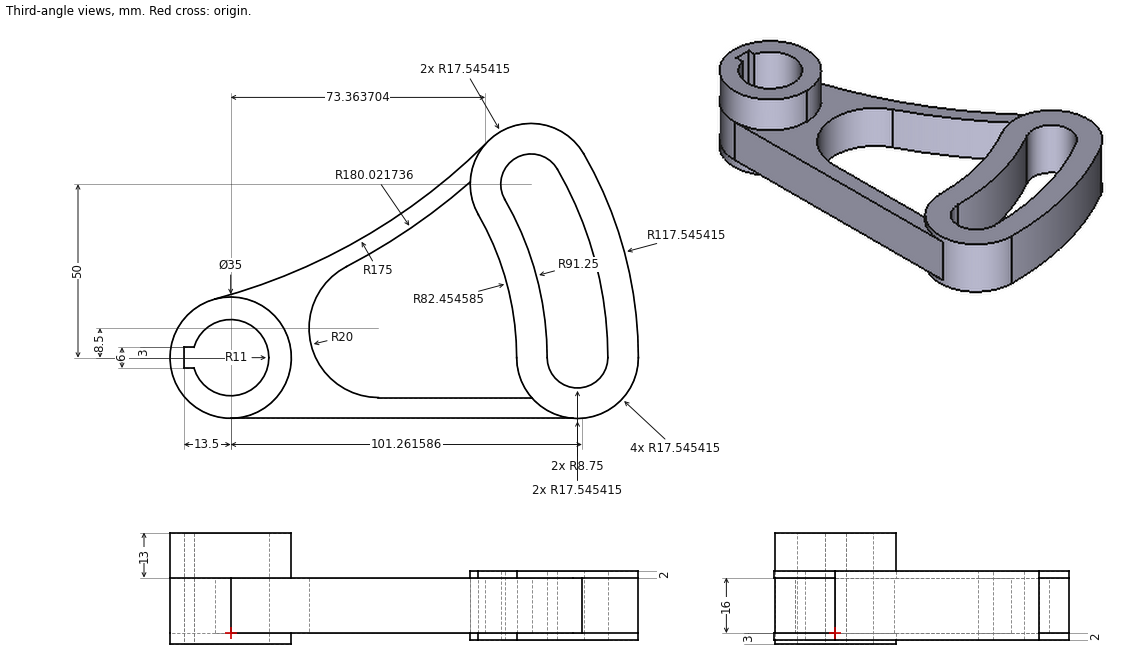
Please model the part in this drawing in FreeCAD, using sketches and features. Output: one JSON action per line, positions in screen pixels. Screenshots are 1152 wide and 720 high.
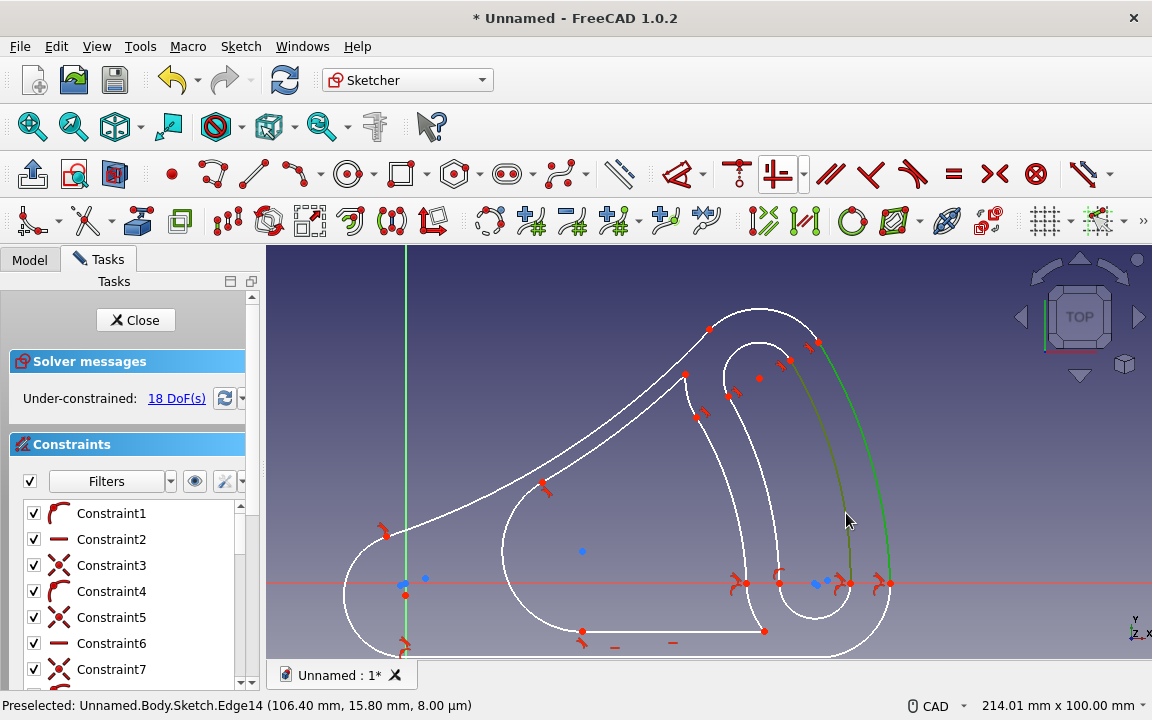
{"action": "left_click", "coordinate": [737, 174]}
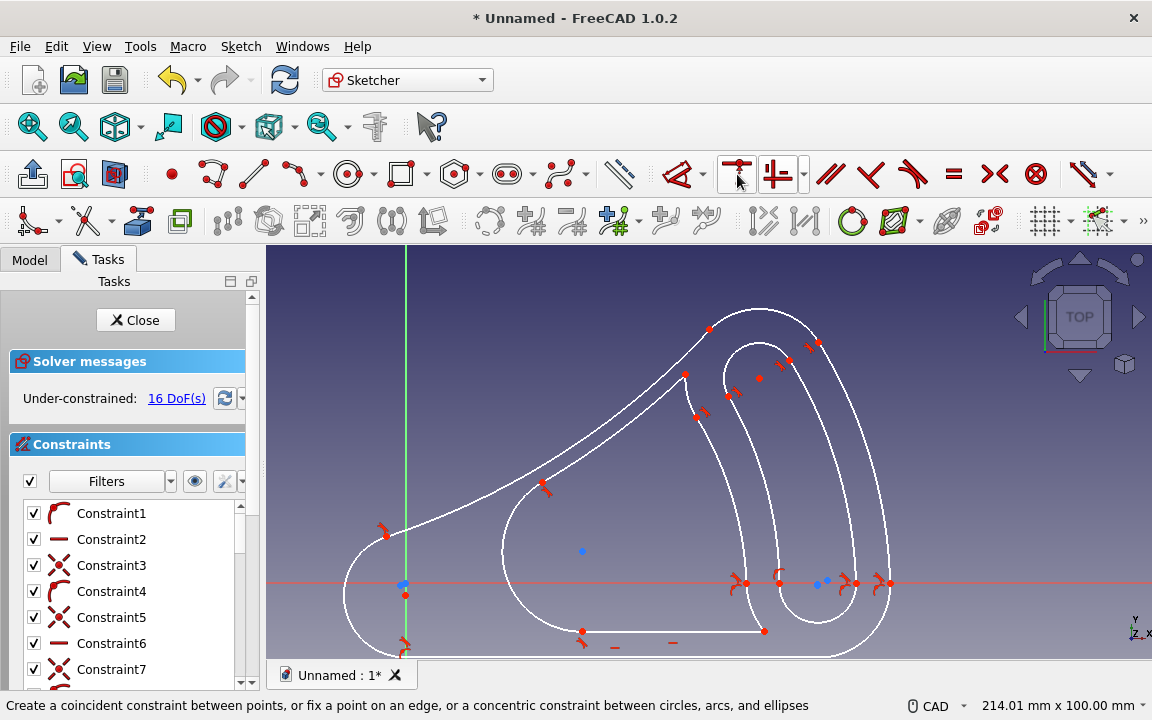
{"action": "left_click", "coordinate": [882, 508]}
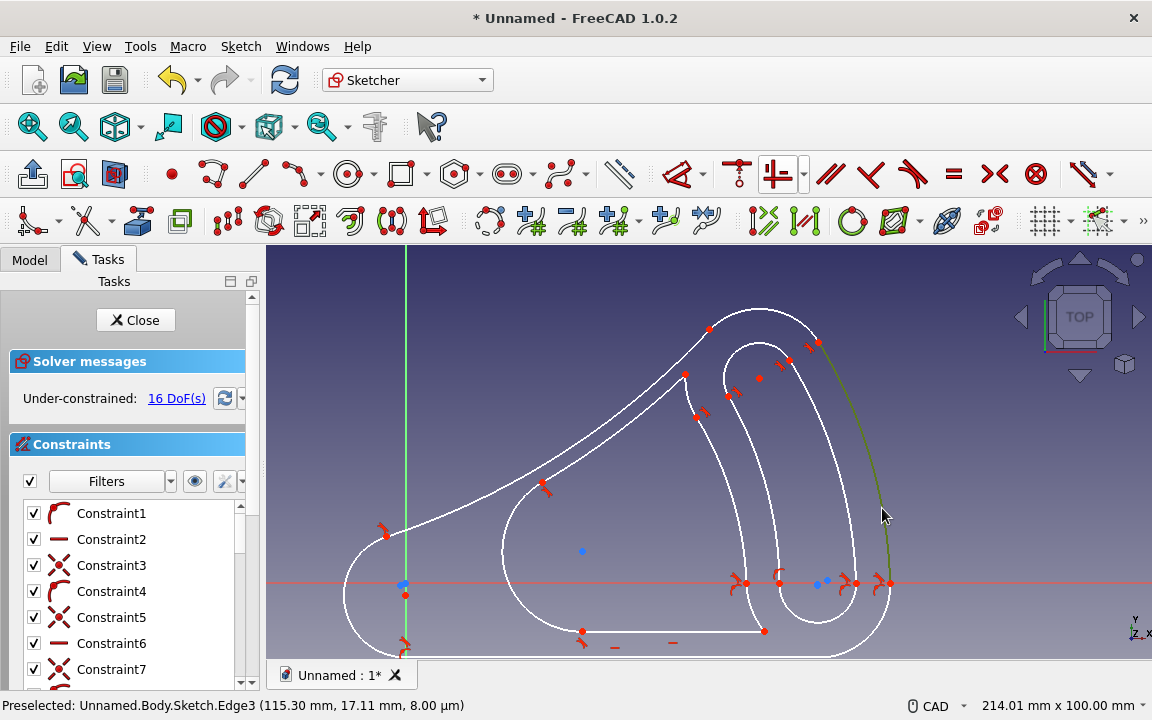
{"action": "left_click", "coordinate": [775, 525]}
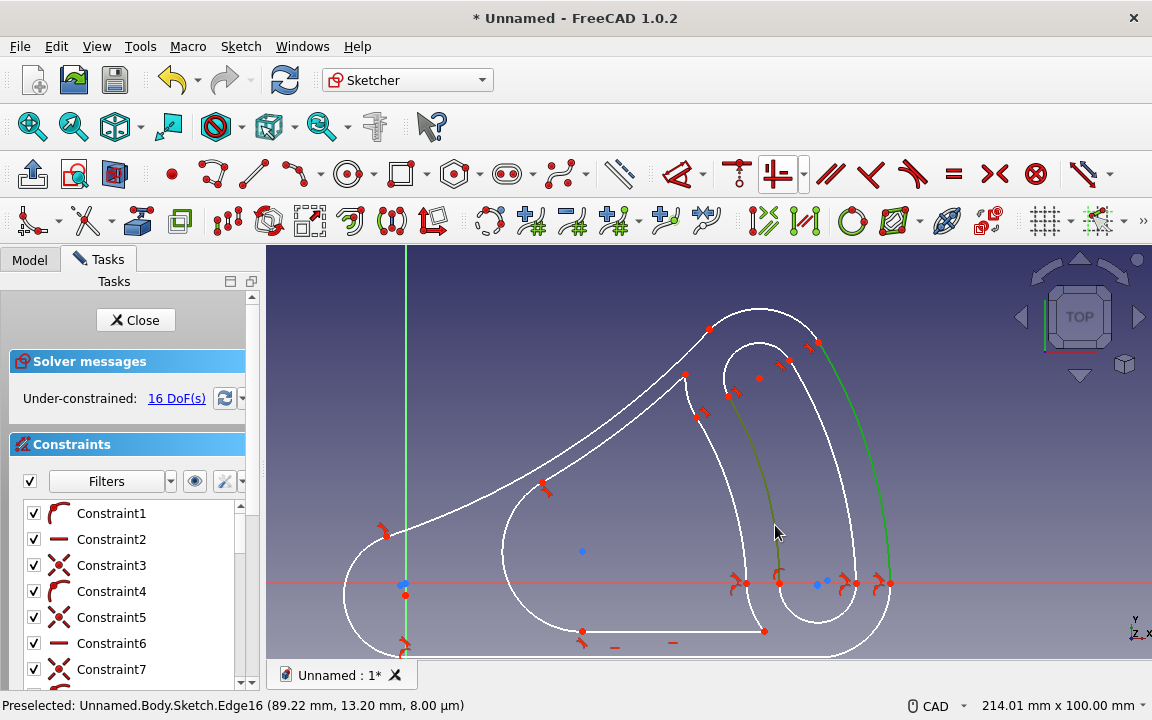
{"action": "left_click", "coordinate": [737, 174]}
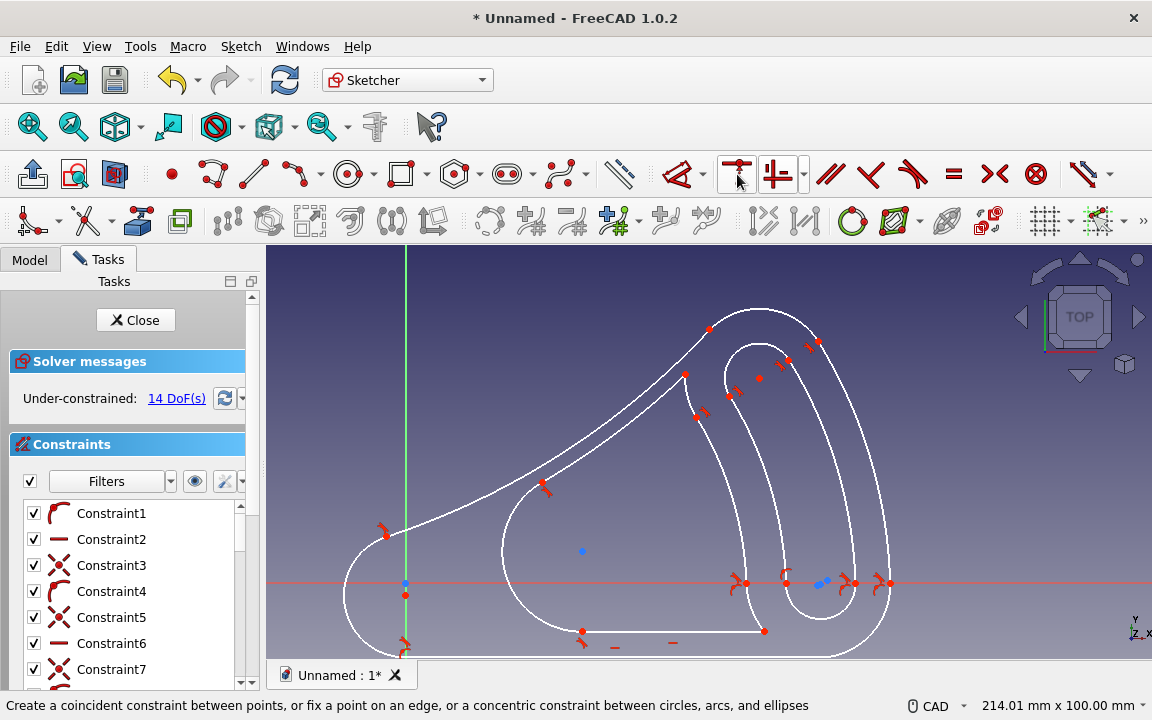
{"action": "left_click", "coordinate": [884, 615]}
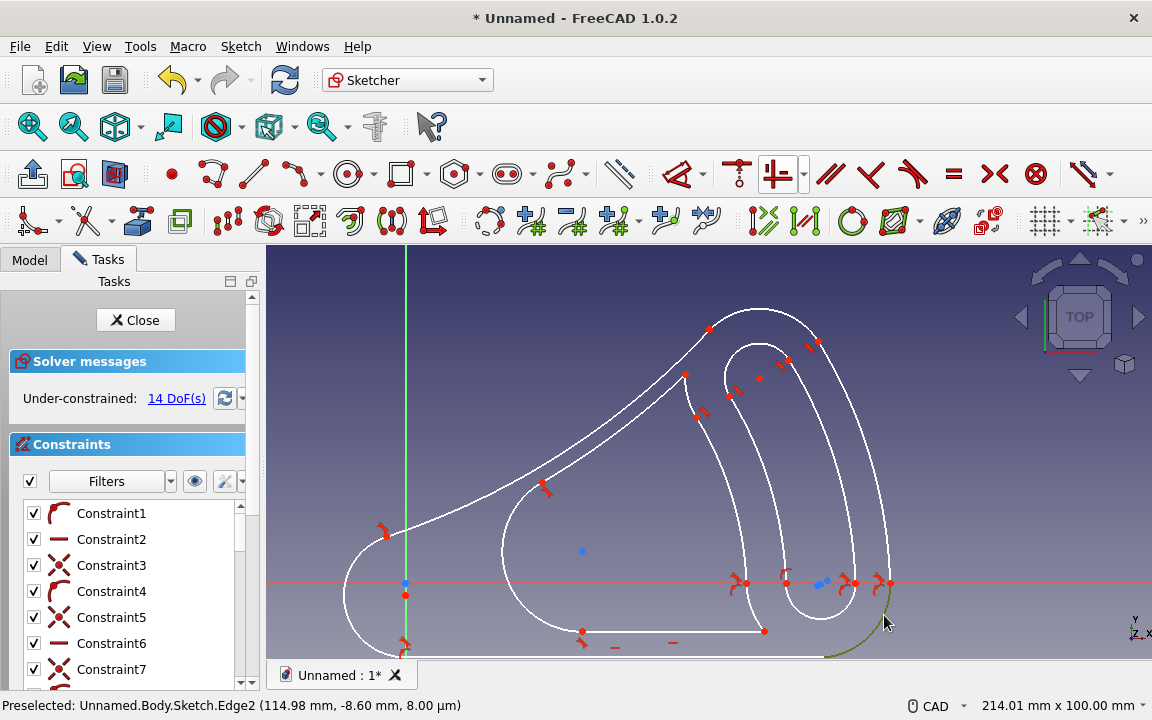
{"action": "left_click", "coordinate": [791, 316]}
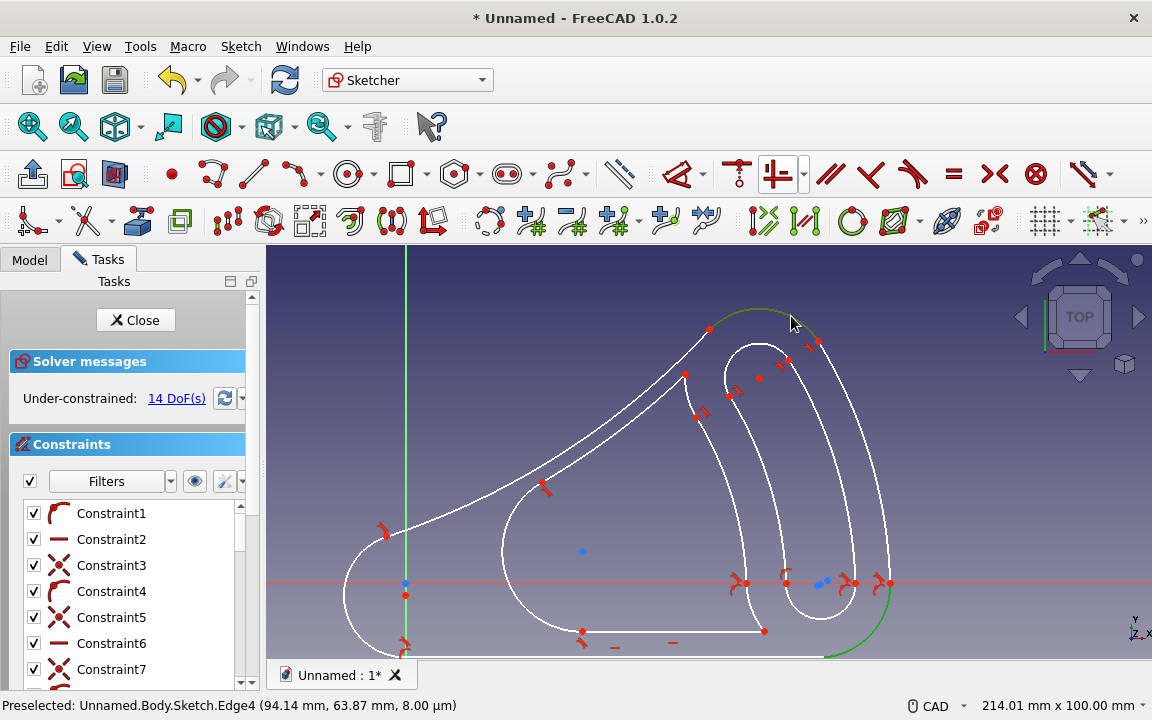
{"action": "scroll", "coordinate": [686, 388], "scroll_direction": "up", "scroll_amount": 2}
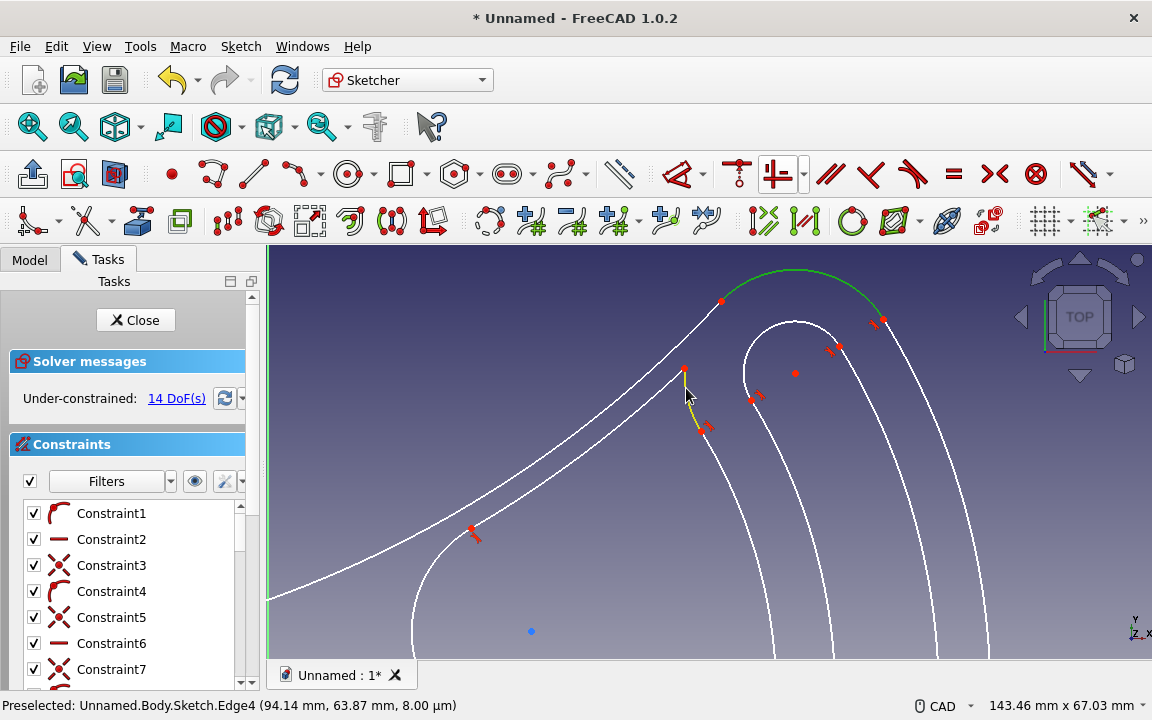
{"action": "left_click", "coordinate": [686, 388]}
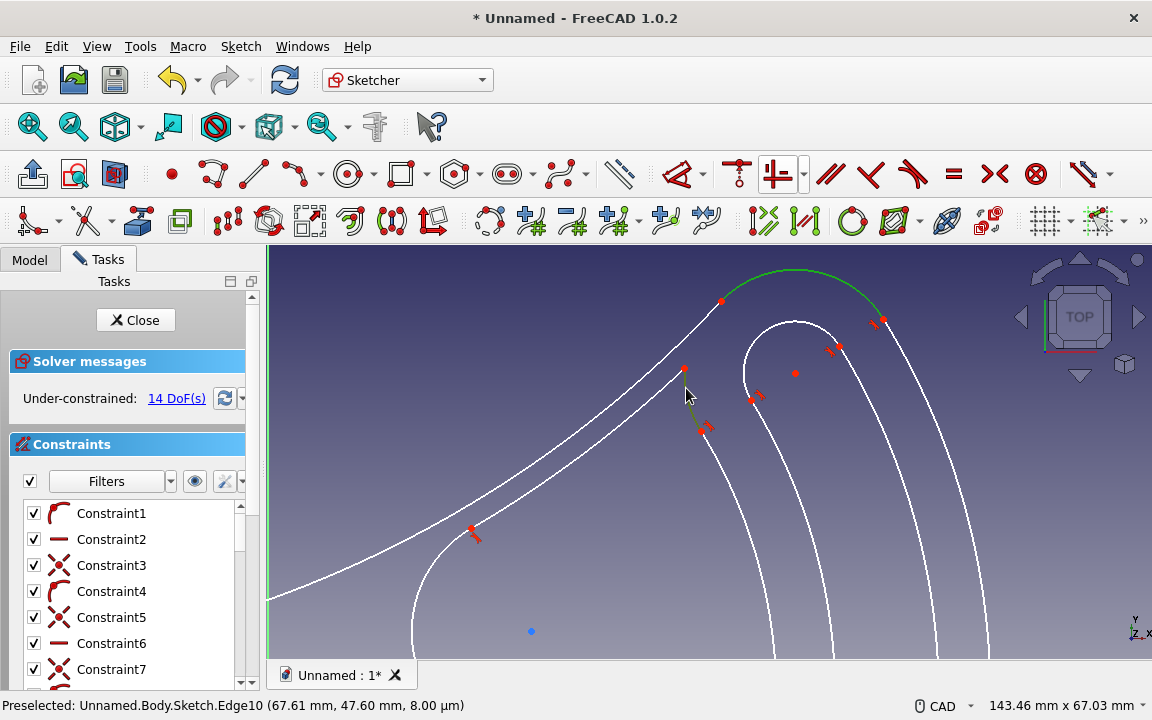
{"action": "scroll", "coordinate": [692, 392], "scroll_direction": "down", "scroll_amount": 4}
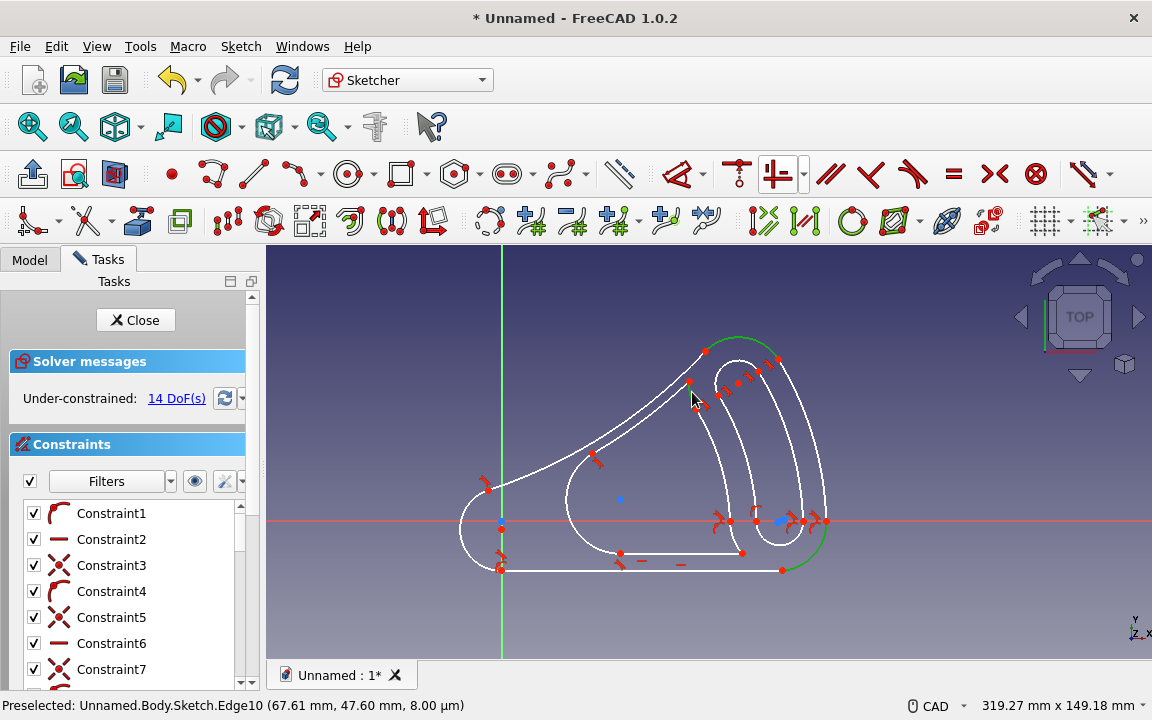
{"action": "scroll", "coordinate": [731, 532], "scroll_direction": "up", "scroll_amount": 2}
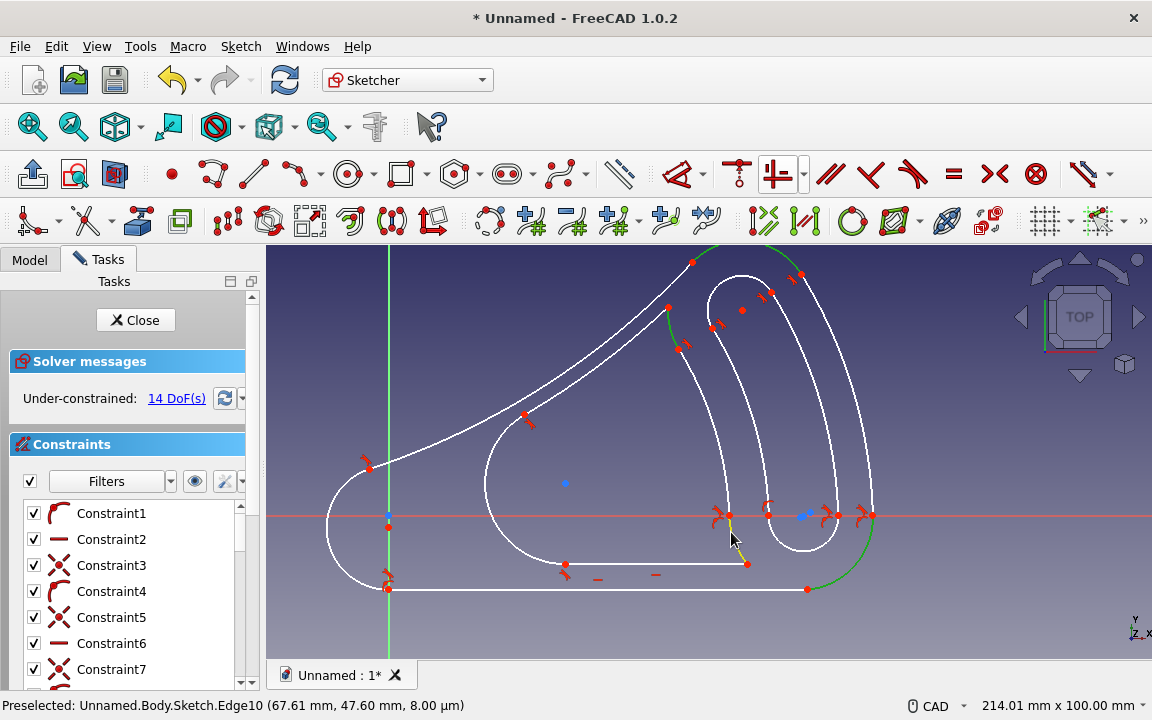
{"action": "left_click", "coordinate": [731, 531]}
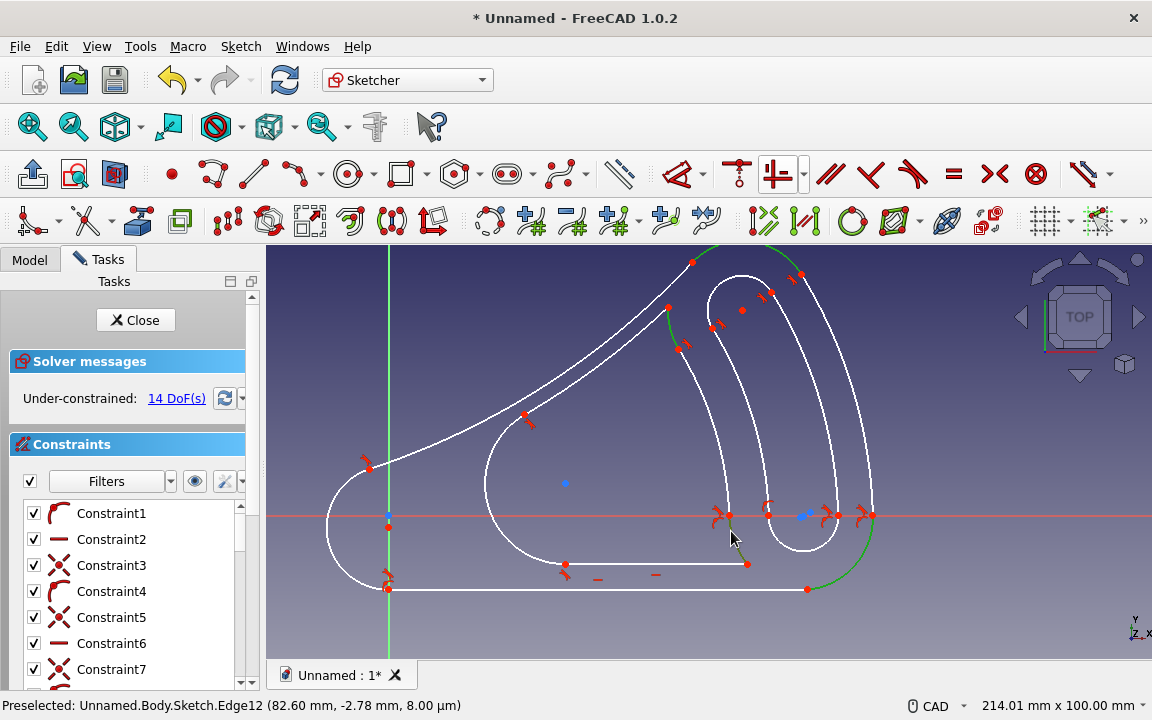
{"action": "left_click", "coordinate": [954, 174]}